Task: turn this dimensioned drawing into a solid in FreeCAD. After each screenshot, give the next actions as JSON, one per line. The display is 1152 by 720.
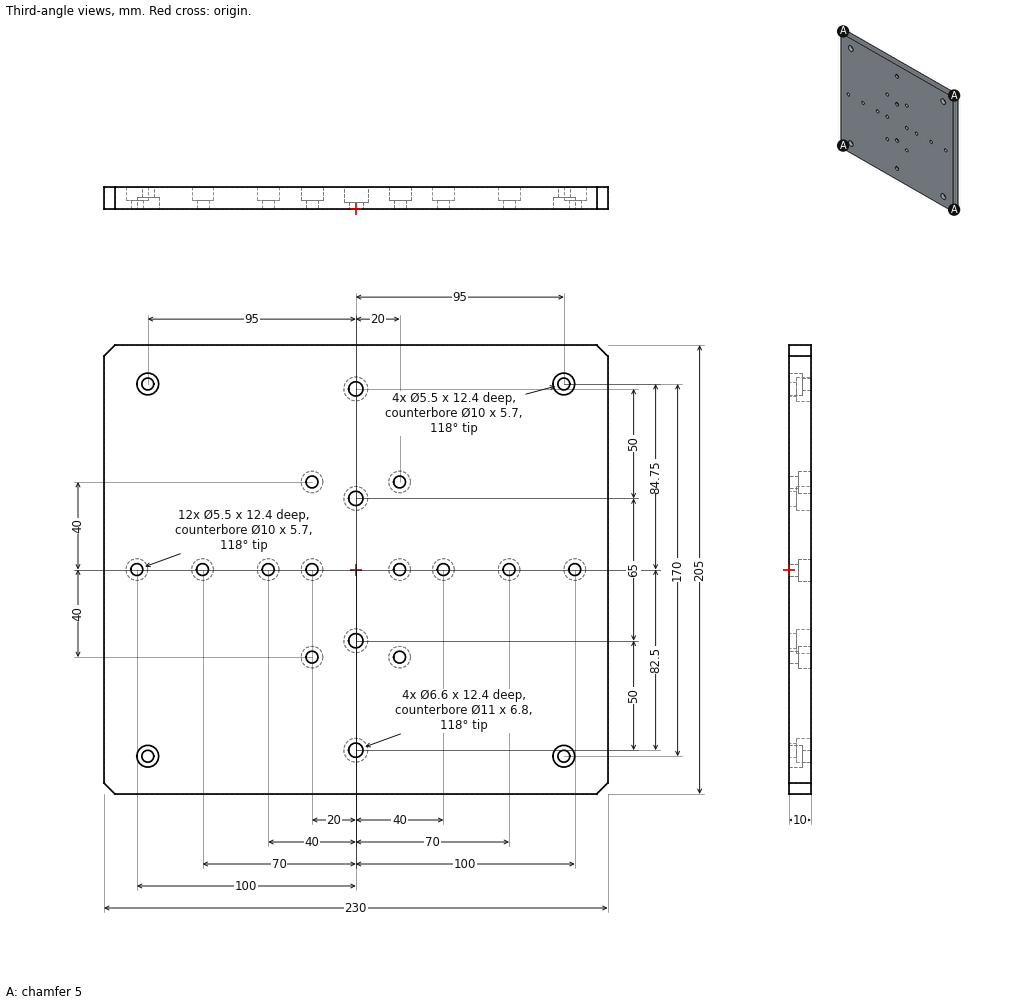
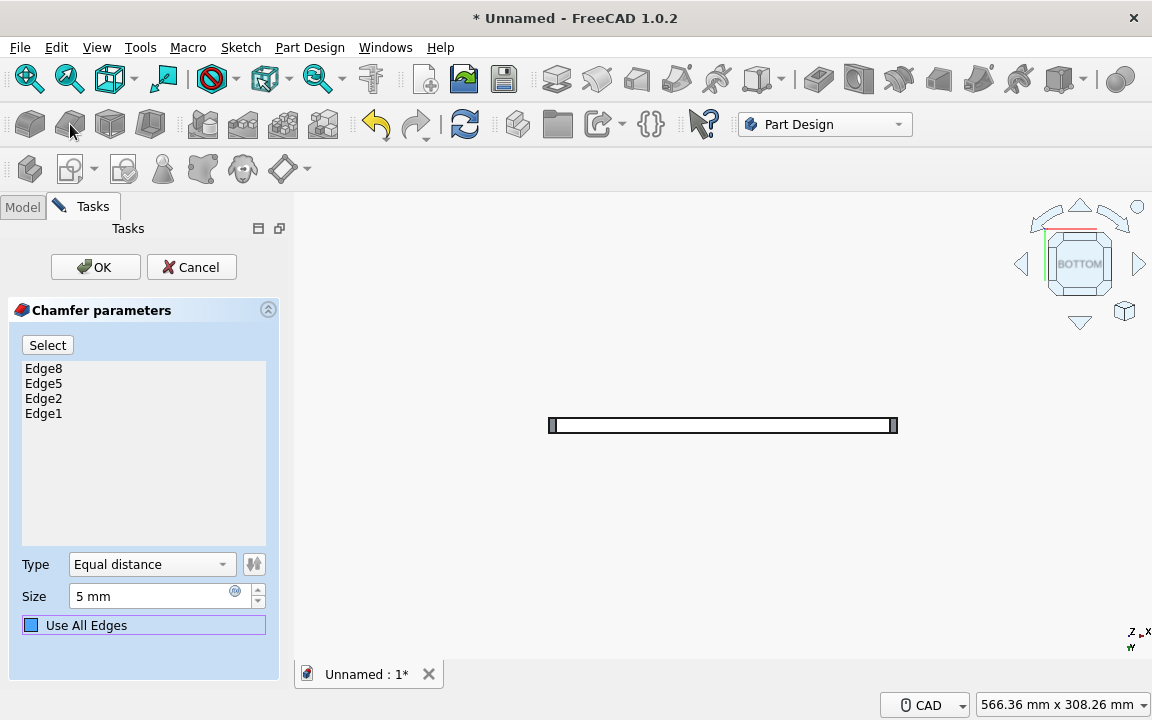
{"action": "left_click", "coordinate": [96, 267]}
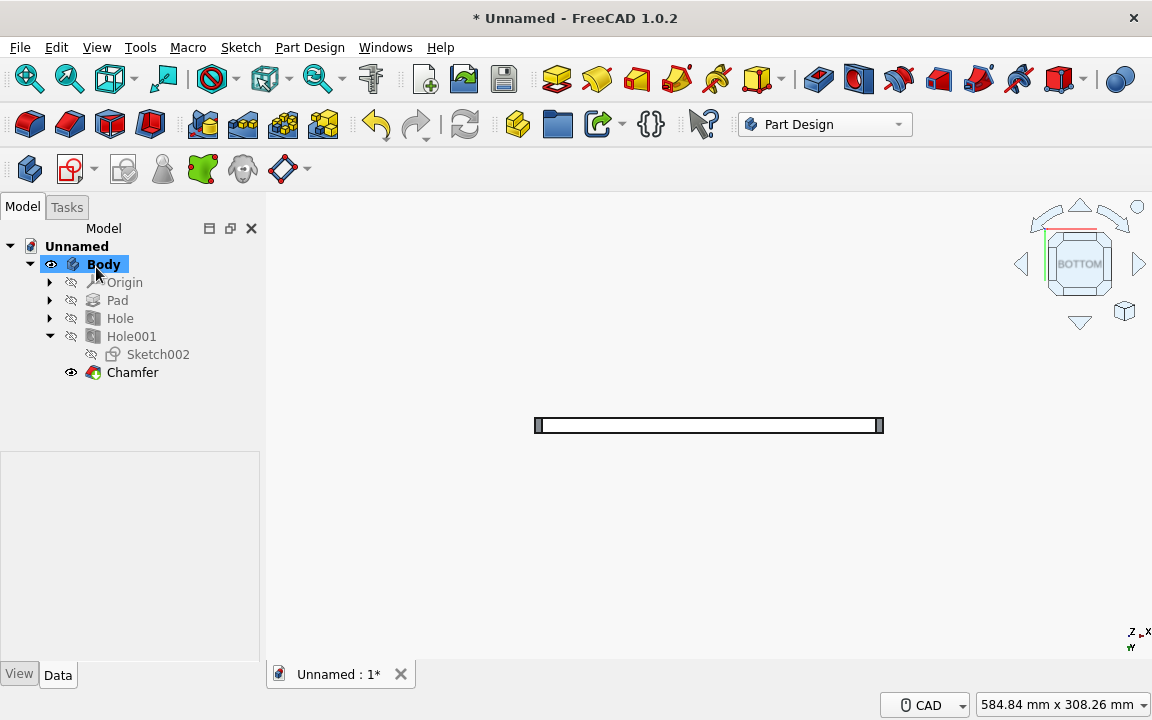
{"action": "left_click", "coordinate": [30, 80]}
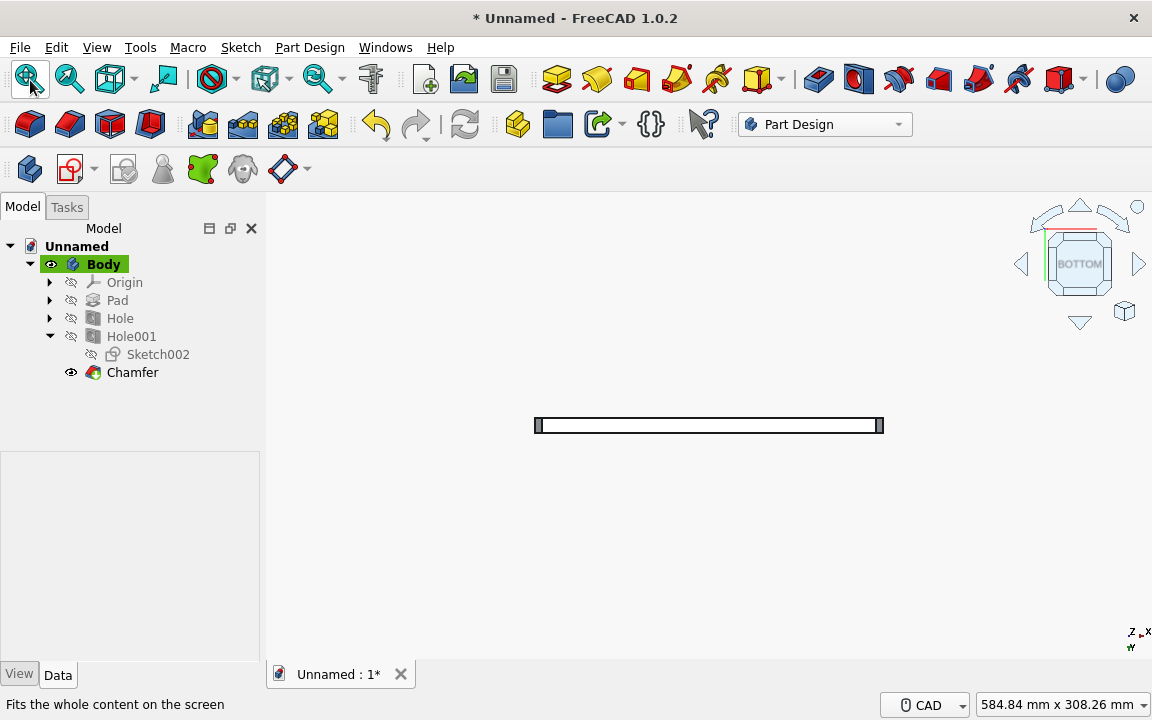
{"action": "key", "text": "4"}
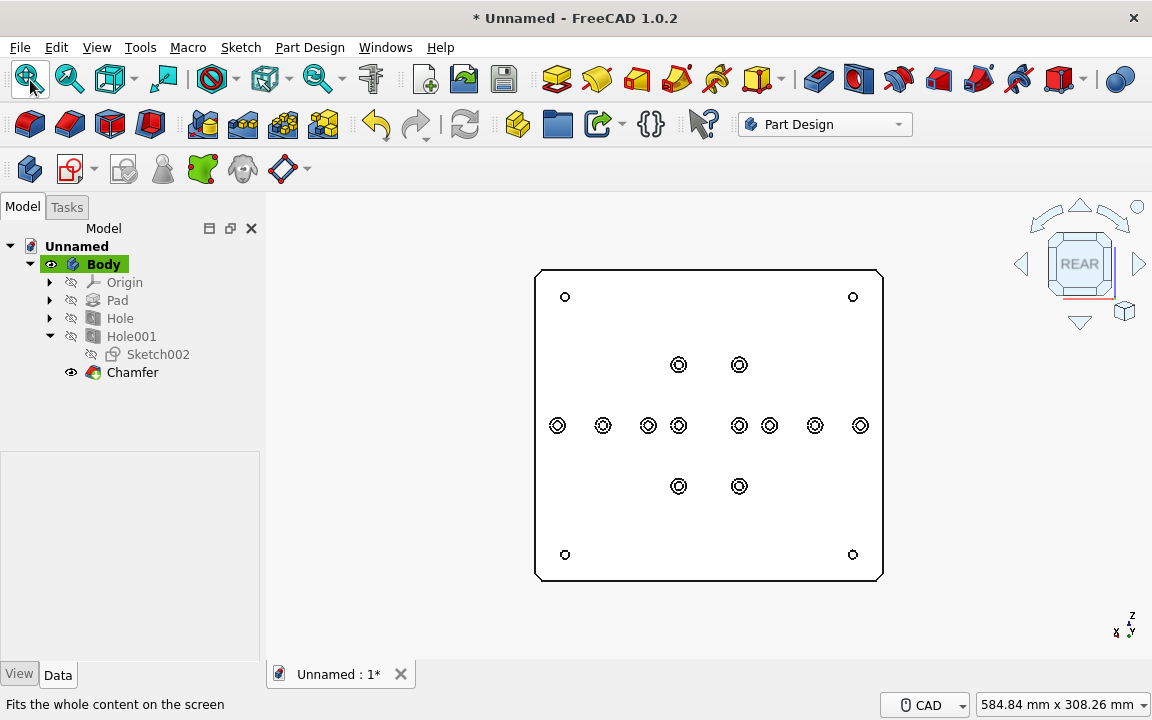
{"action": "left_click", "coordinate": [809, 513]}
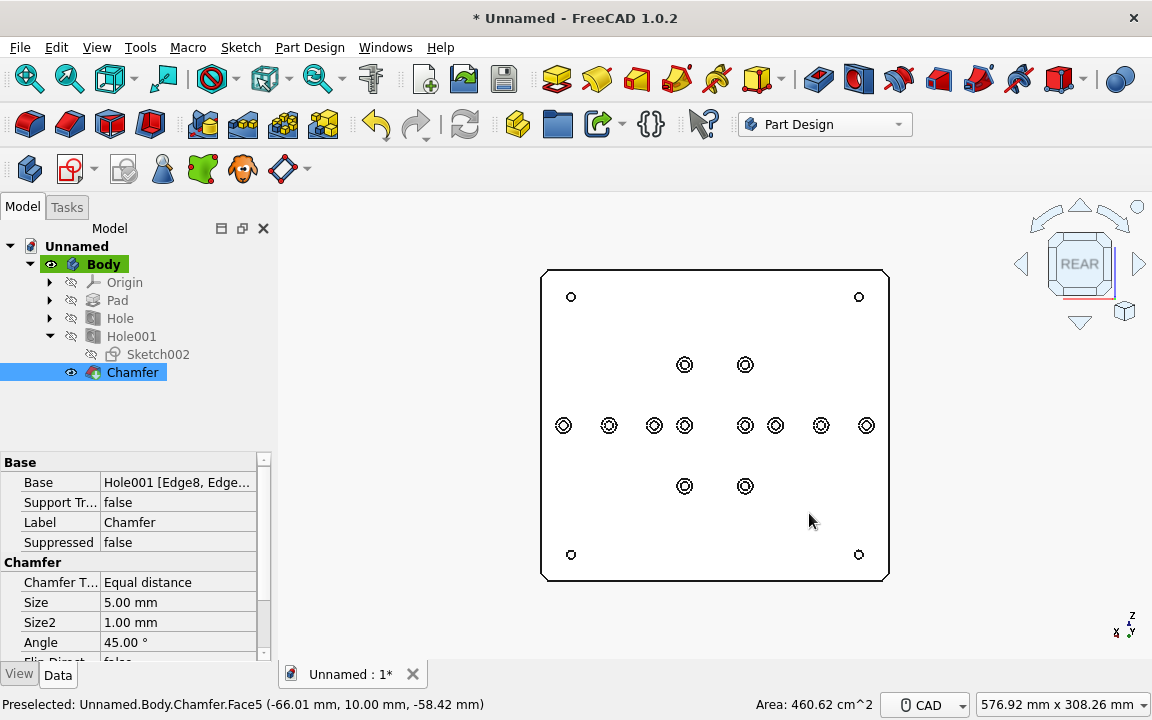
{"action": "left_click", "coordinate": [70, 170]}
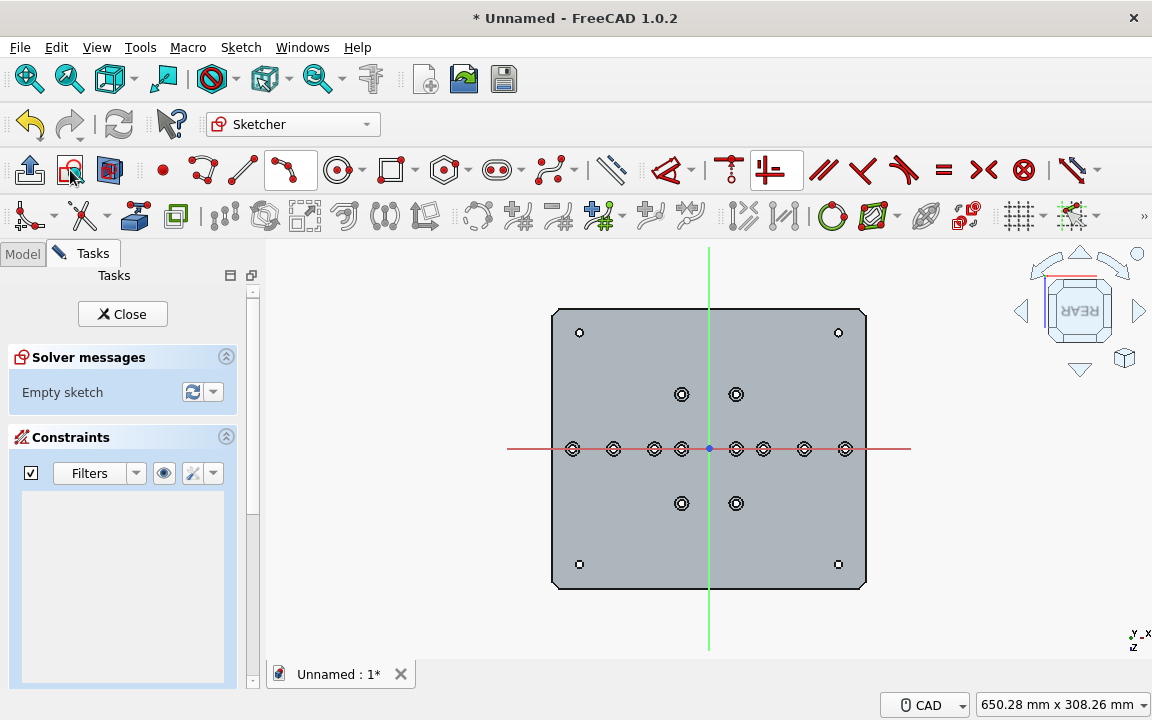
{"action": "left_click", "coordinate": [338, 170]}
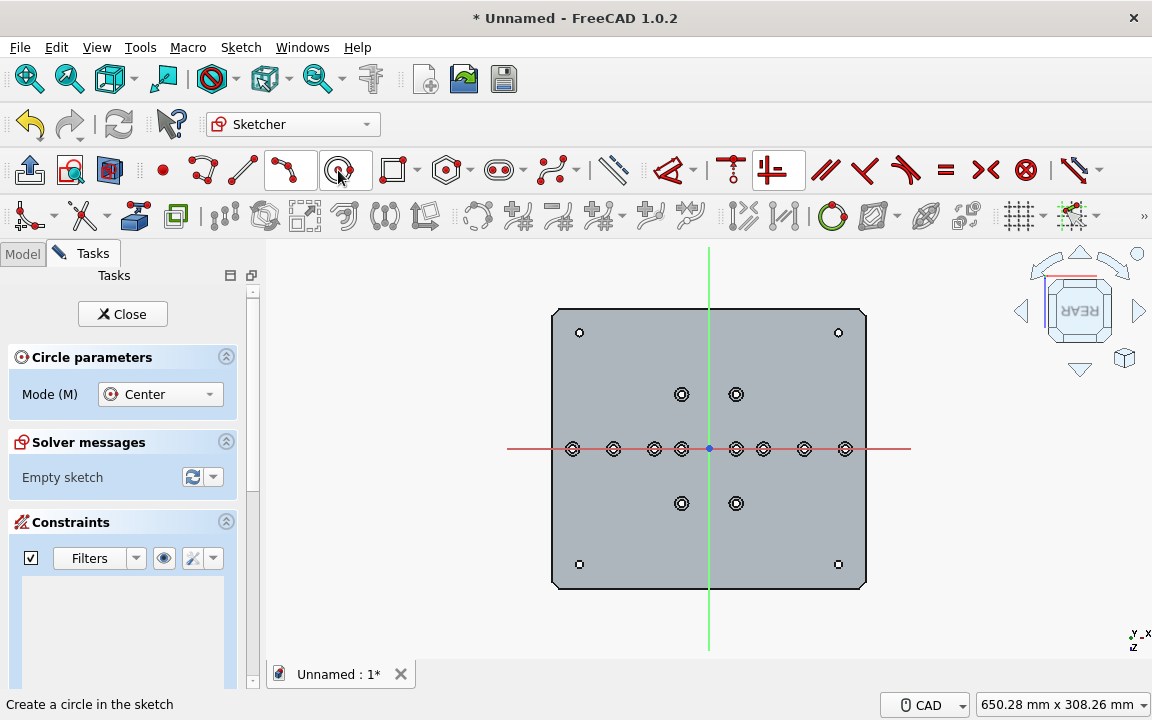
{"action": "scroll", "coordinate": [709, 337], "scroll_direction": "up", "scroll_amount": 9}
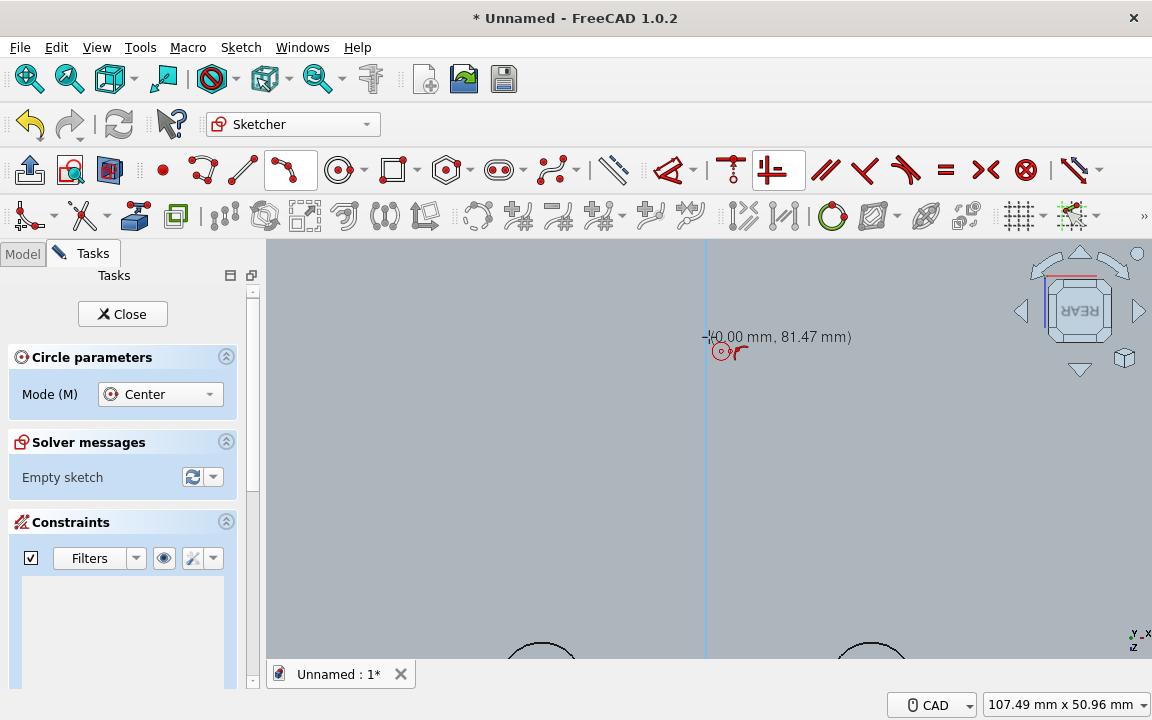
{"action": "scroll", "coordinate": [627, 337], "scroll_direction": "down", "scroll_amount": 9}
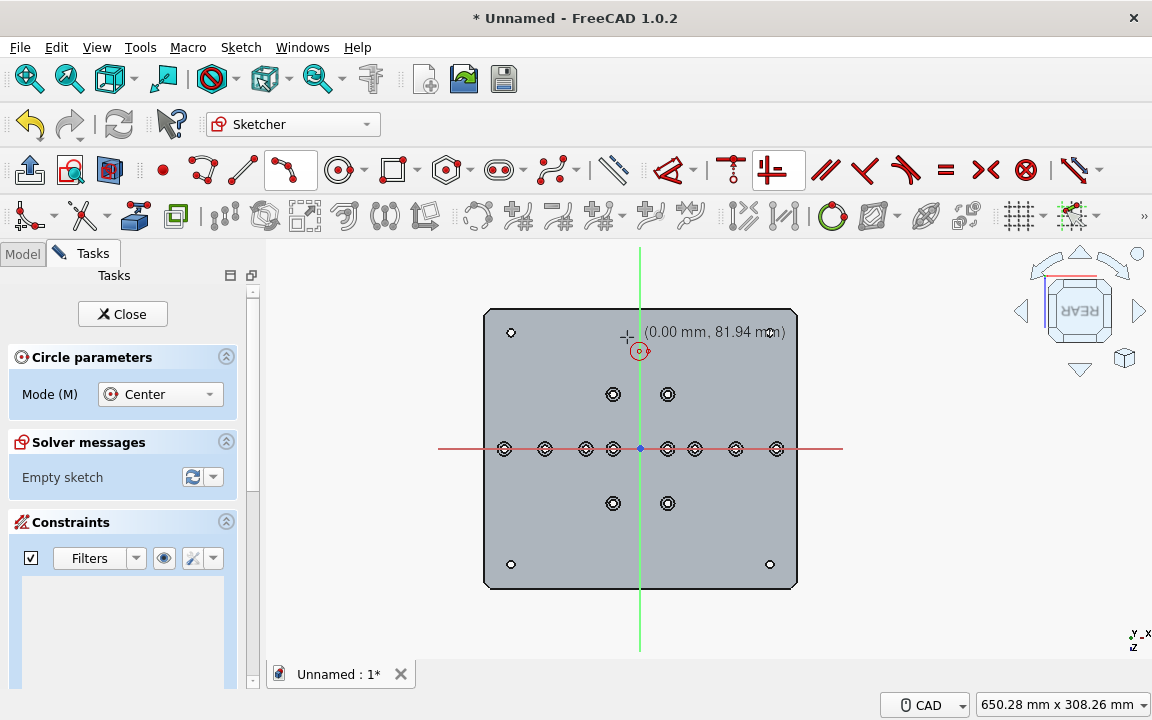
{"action": "left_click", "coordinate": [640, 337]}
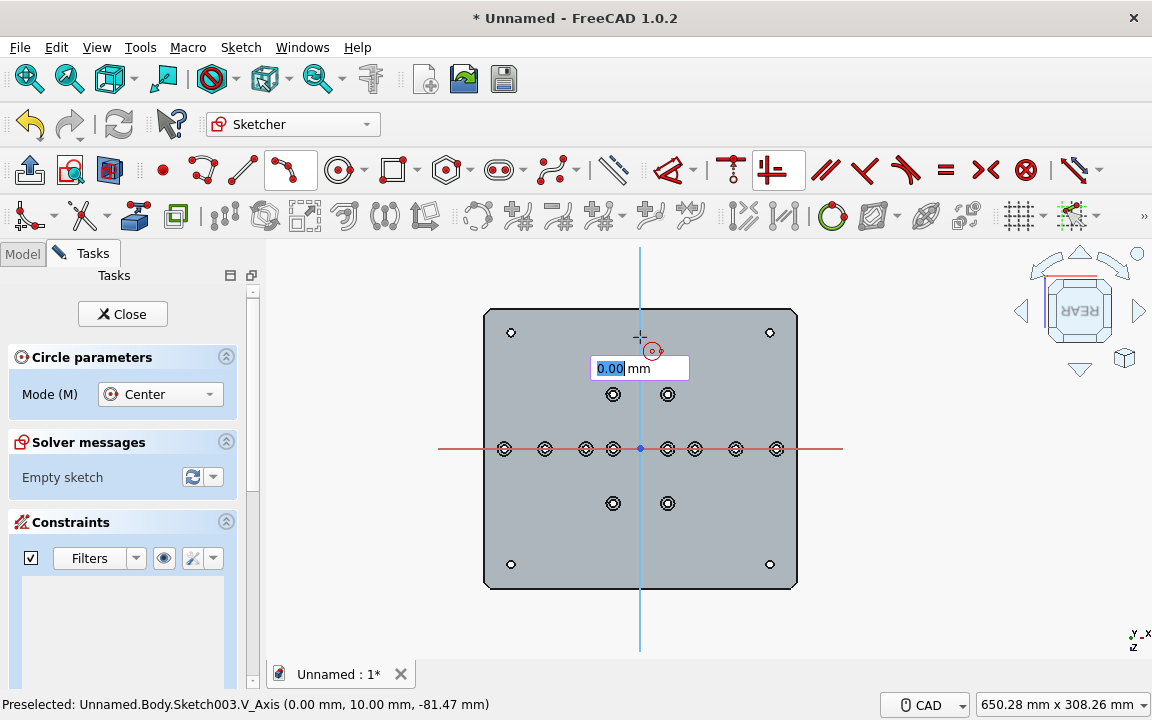
{"action": "scroll", "coordinate": [645, 335], "scroll_direction": "up", "scroll_amount": 7}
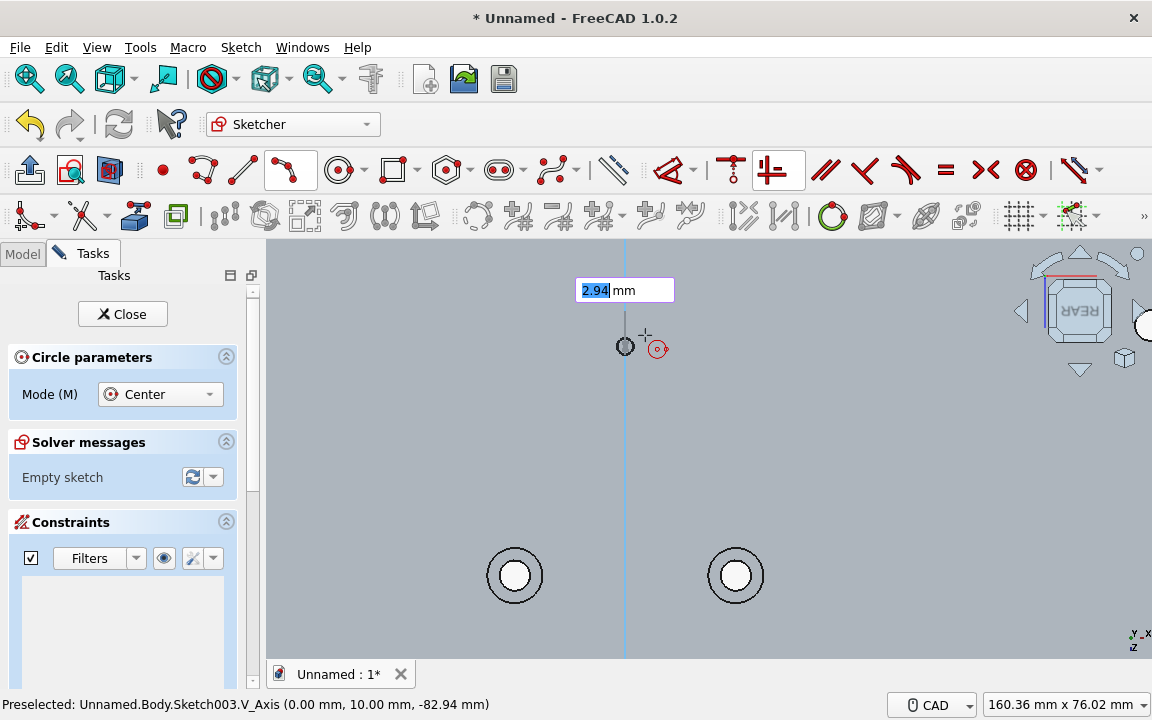
{"action": "left_click", "coordinate": [642, 335]}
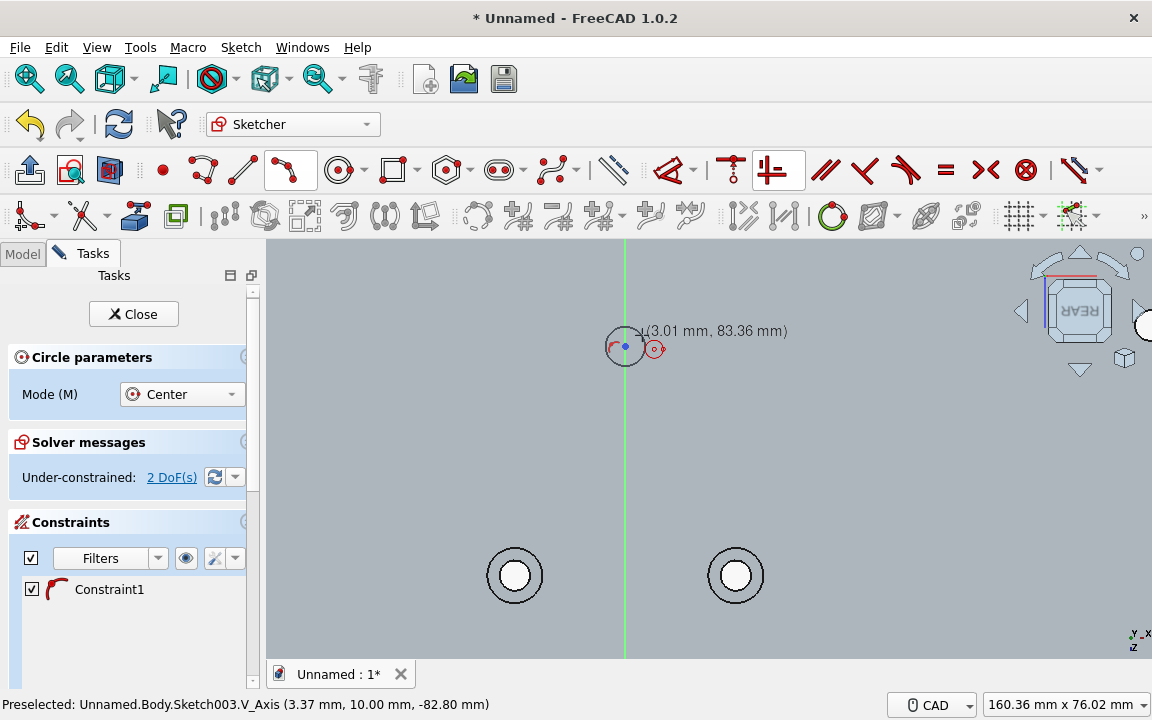
{"action": "scroll", "coordinate": [625, 617], "scroll_direction": "up", "scroll_amount": 2}